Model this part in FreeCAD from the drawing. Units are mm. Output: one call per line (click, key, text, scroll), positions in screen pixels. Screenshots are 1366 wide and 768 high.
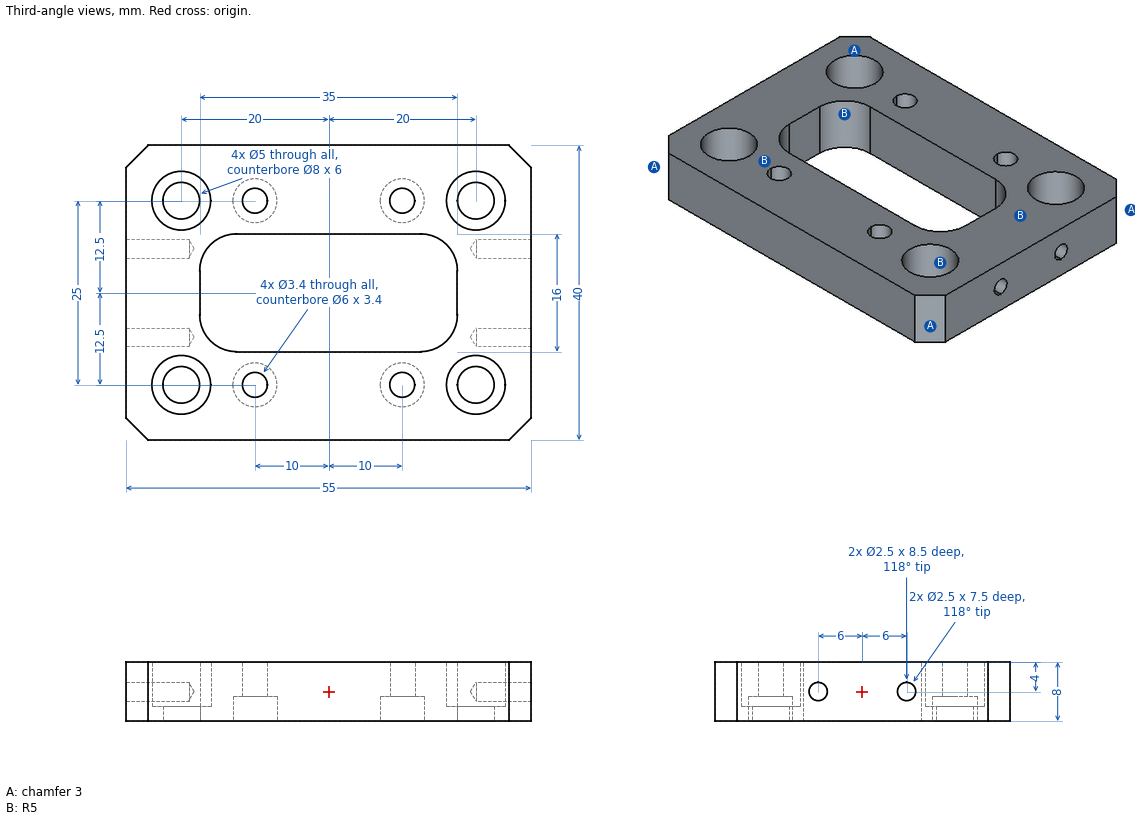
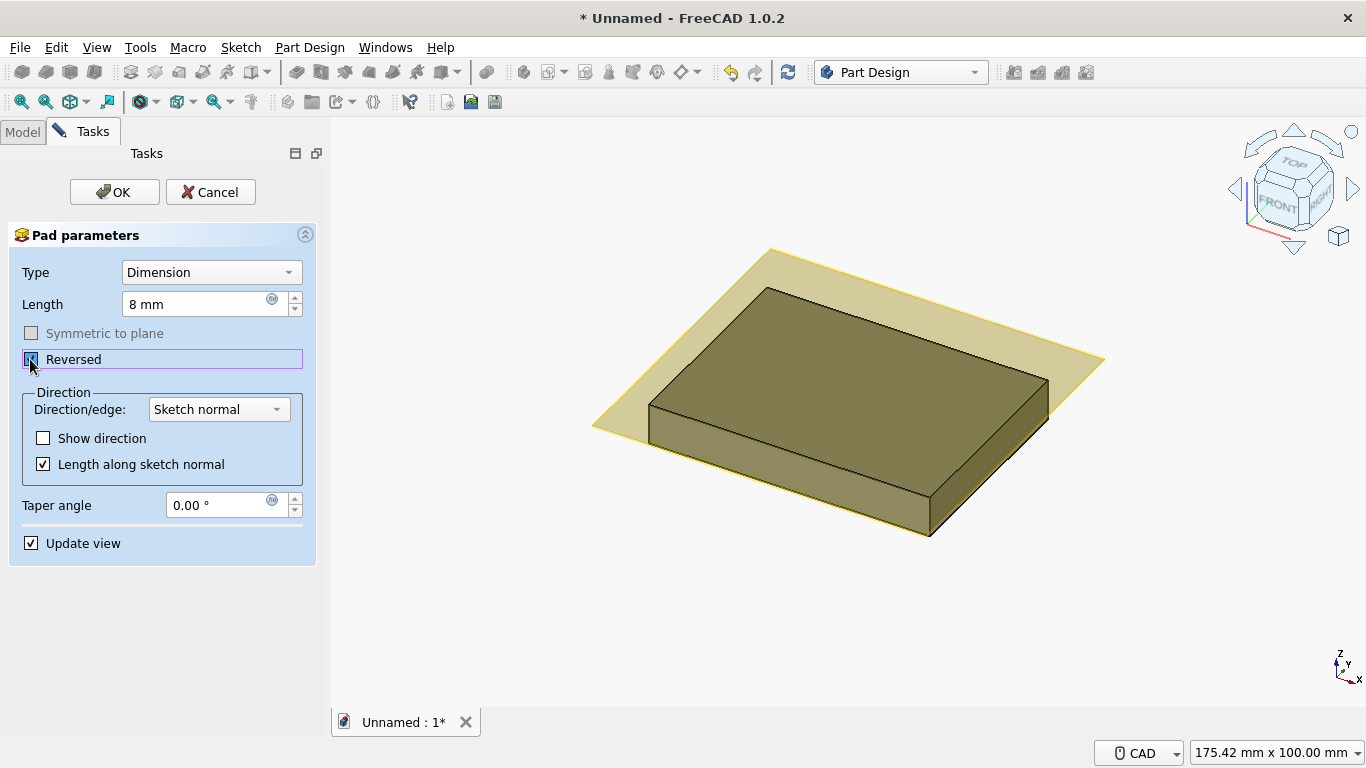
click(115, 192)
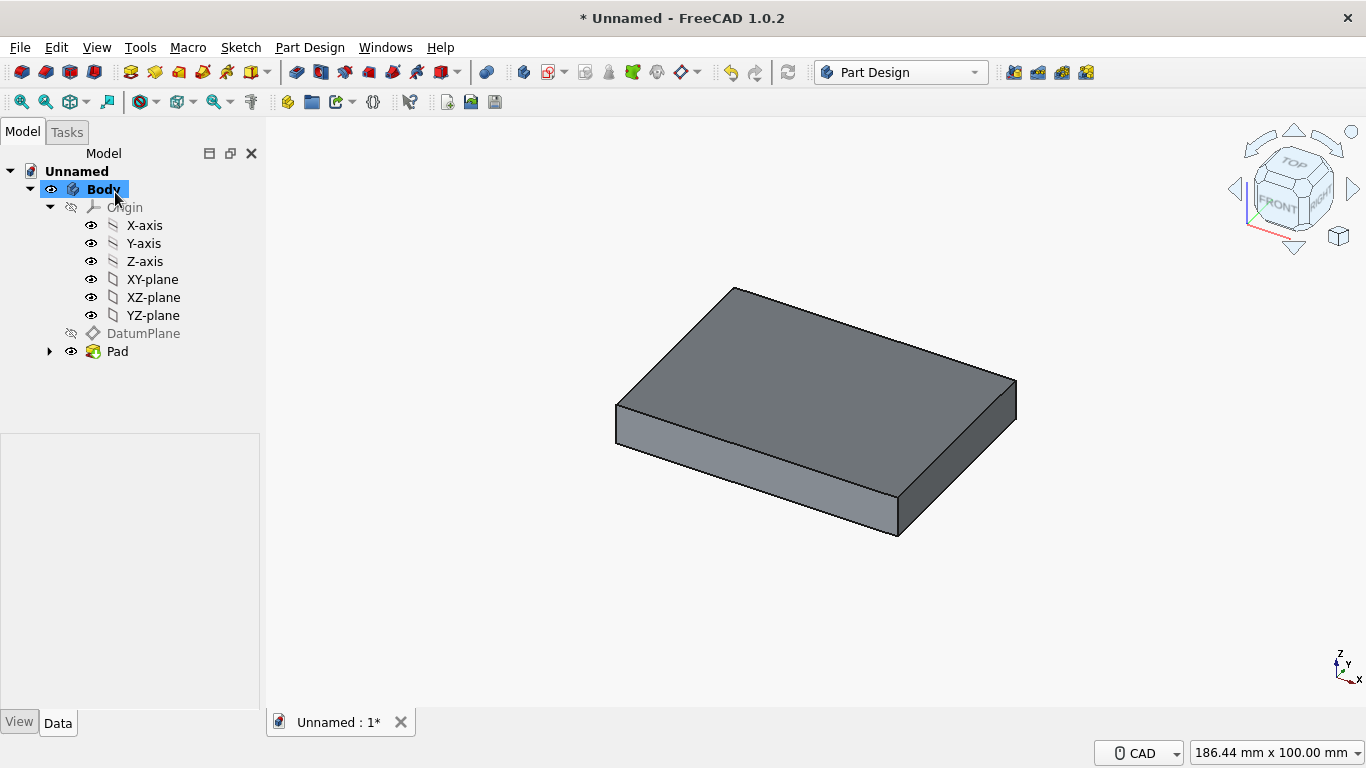
click(22, 102)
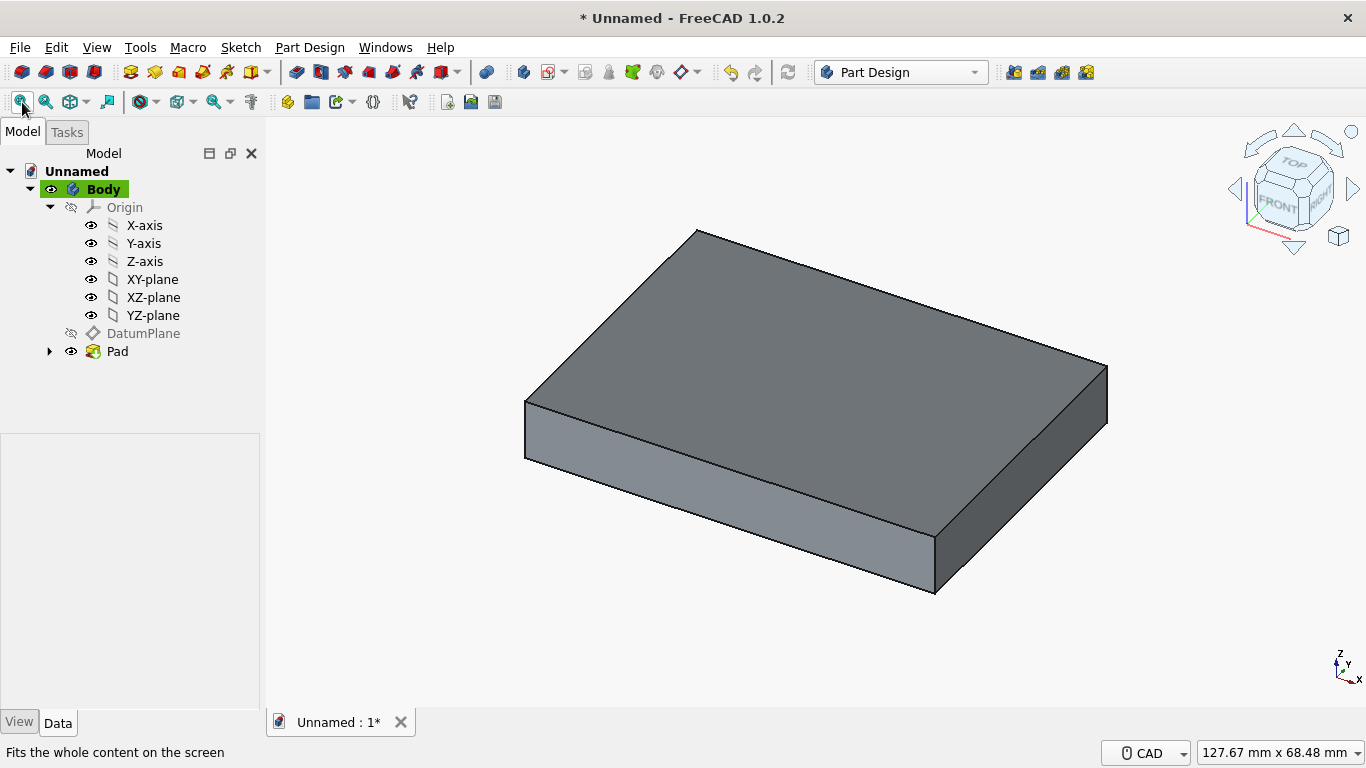
key(5)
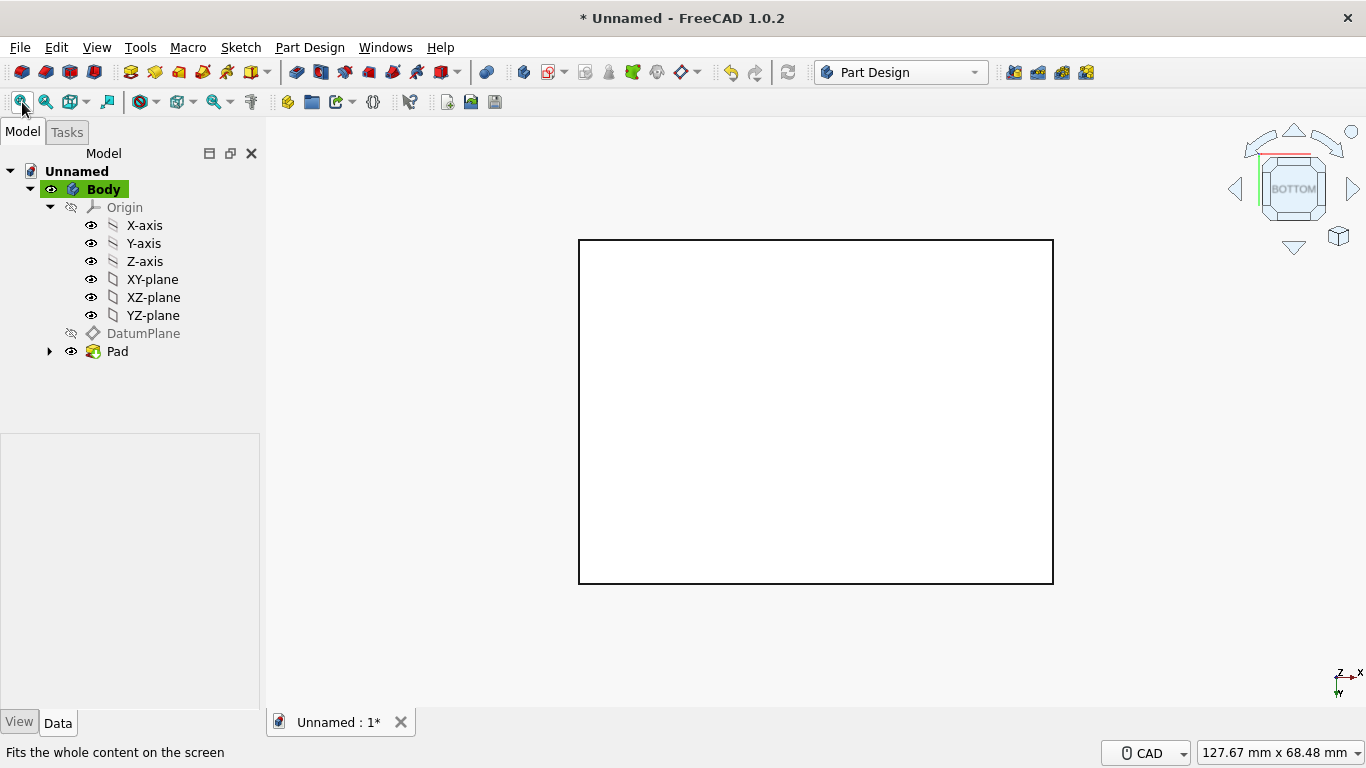
click(816, 411)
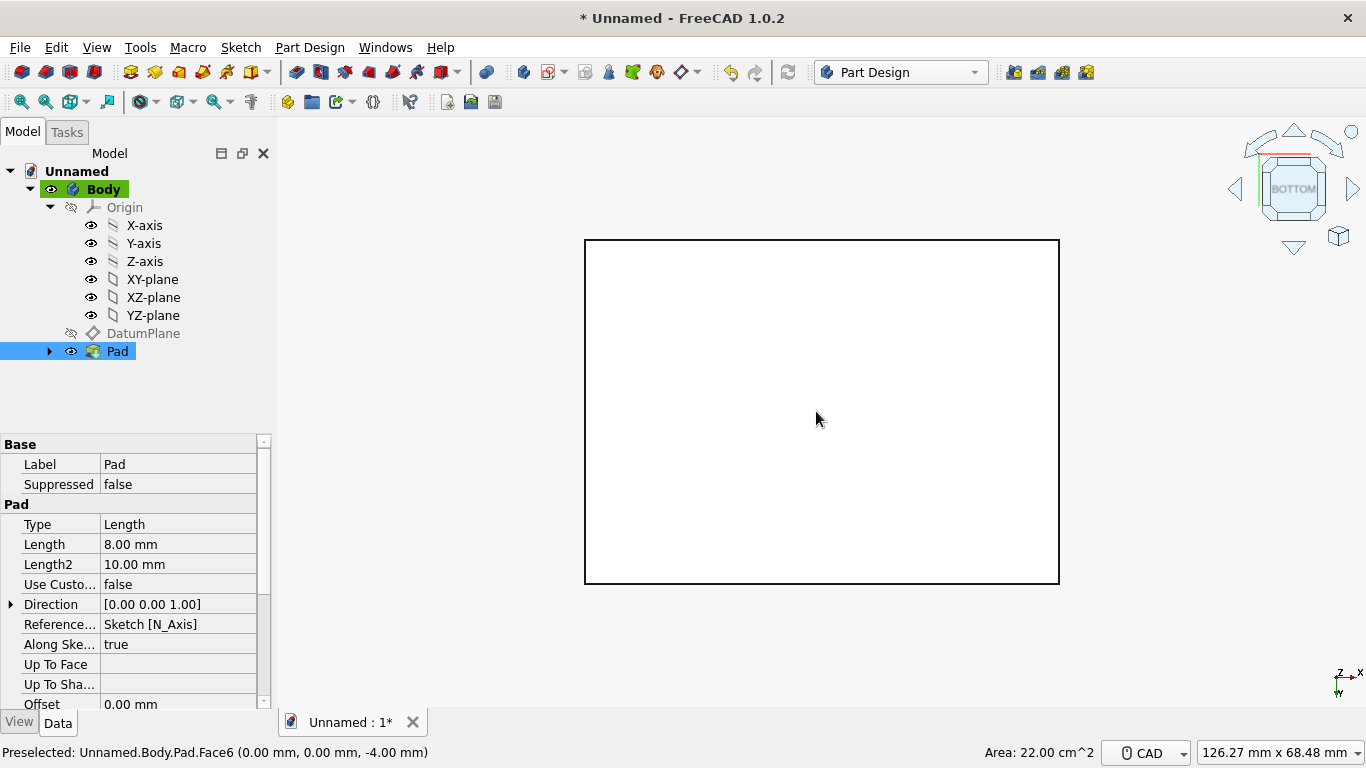
click(548, 72)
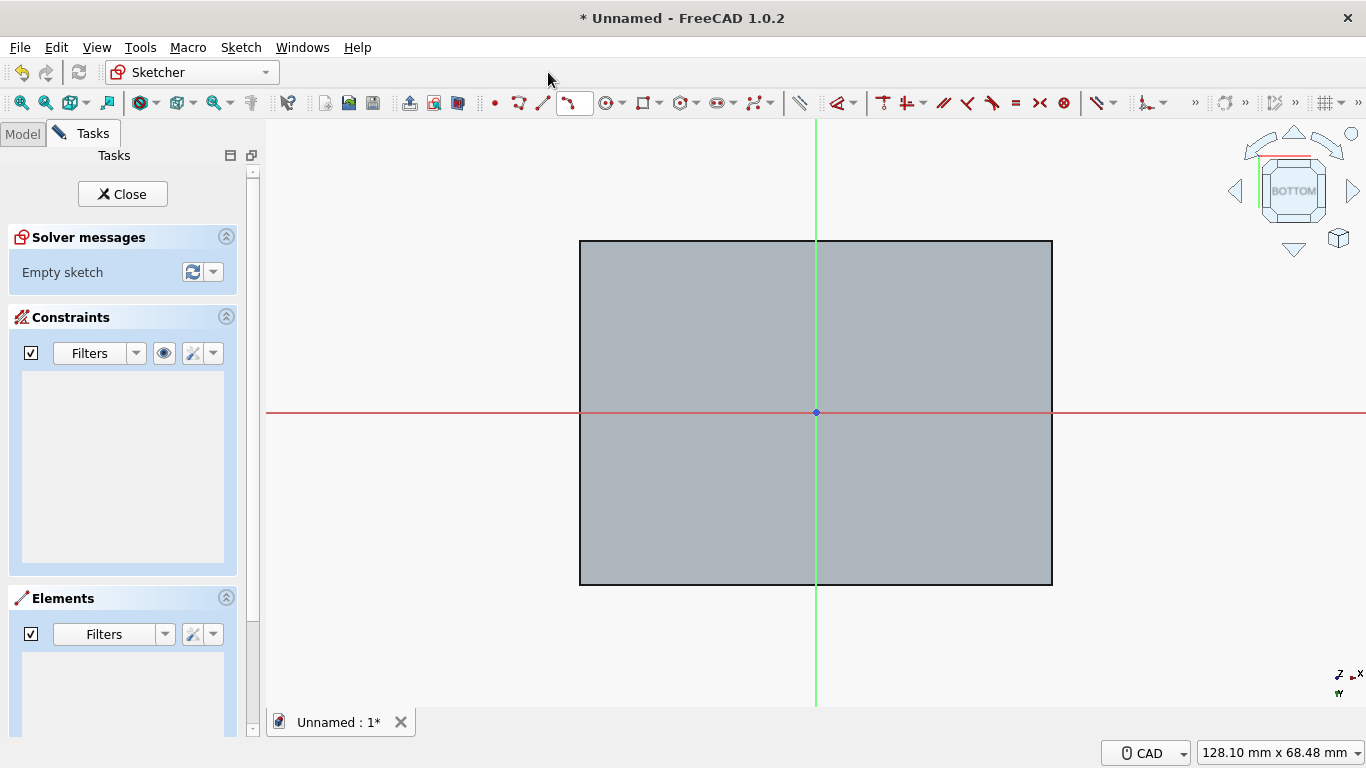
scroll(872, 413, up, 4)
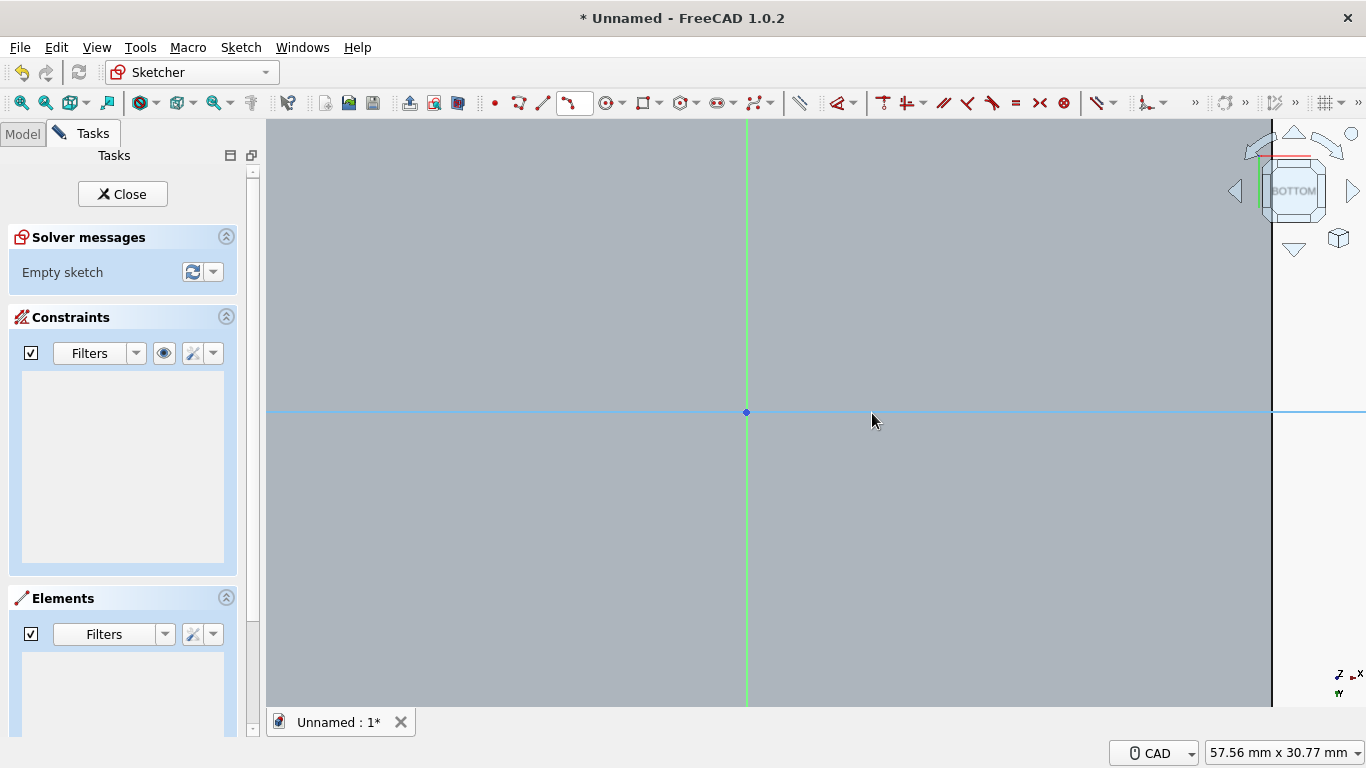
click(662, 104)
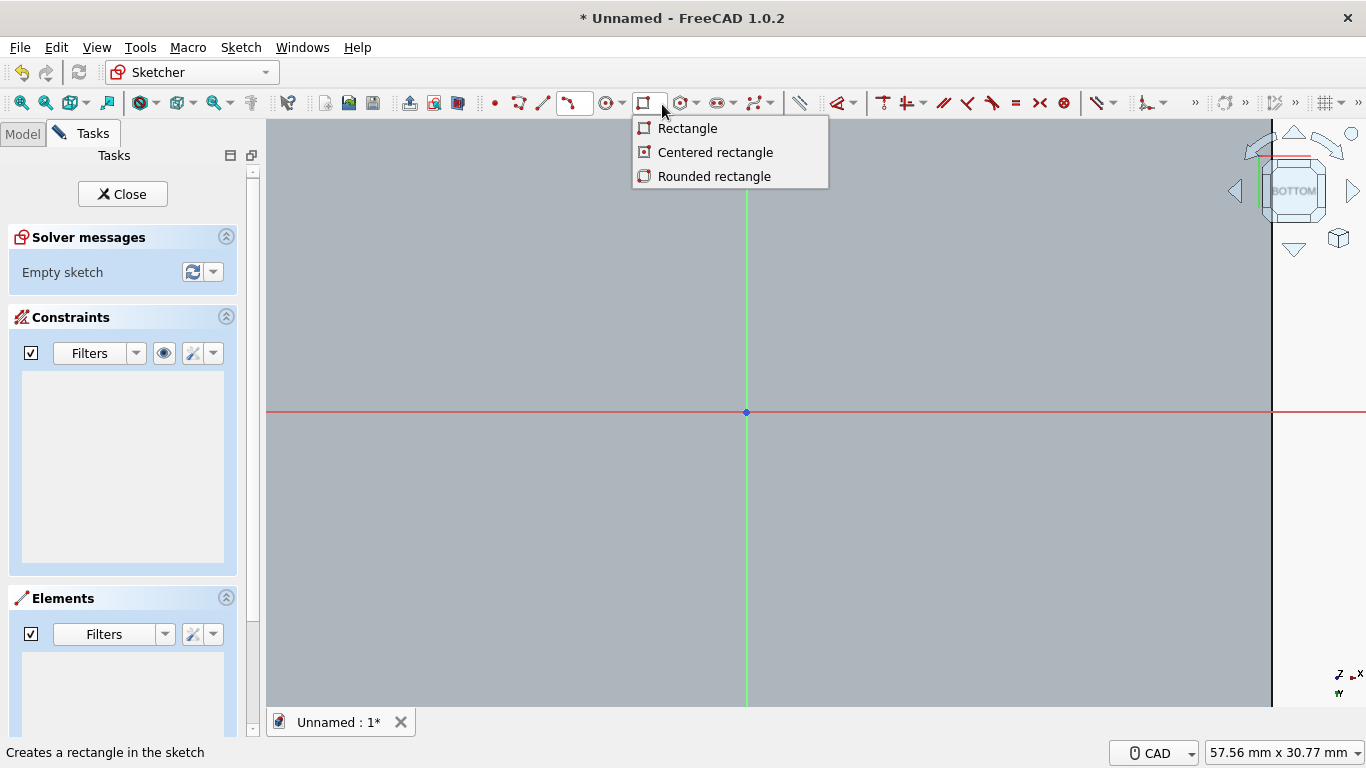
click(730, 152)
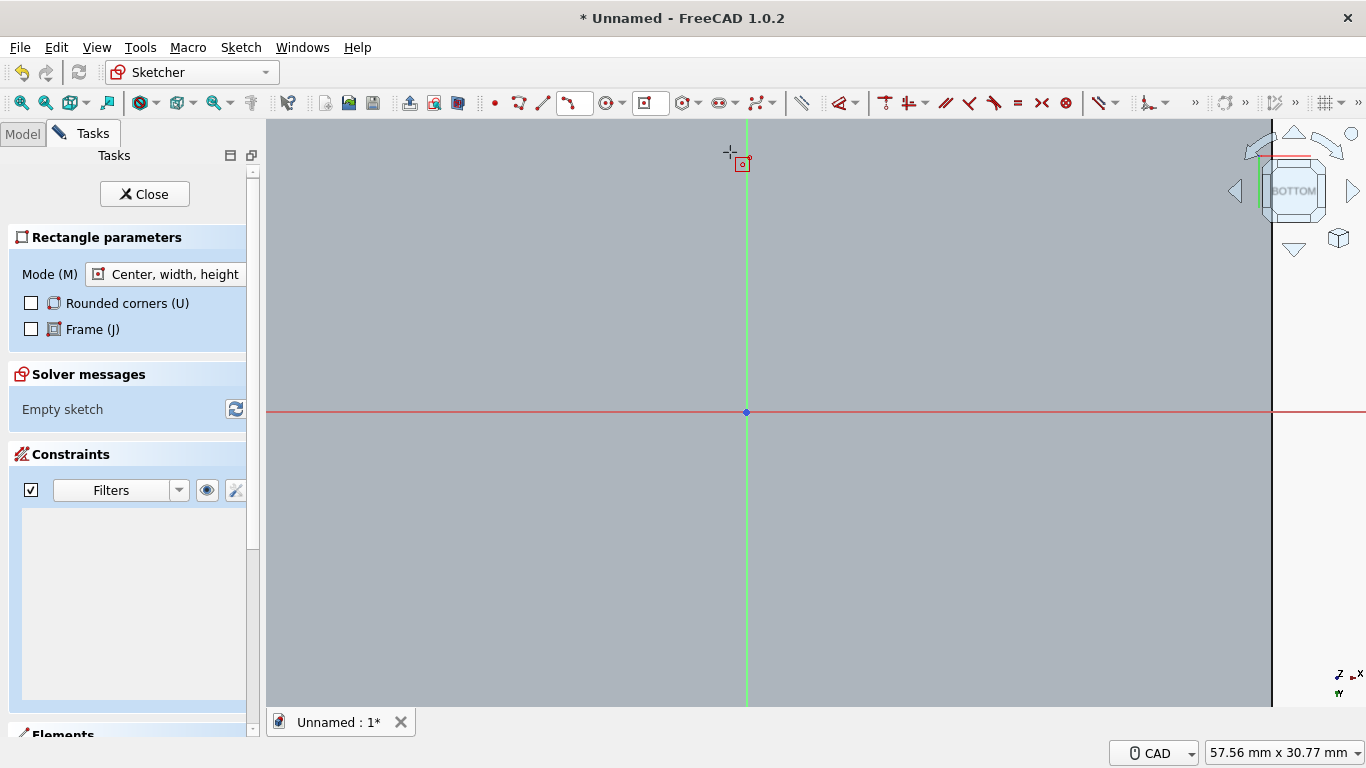
click(747, 412)
move(1081, 260)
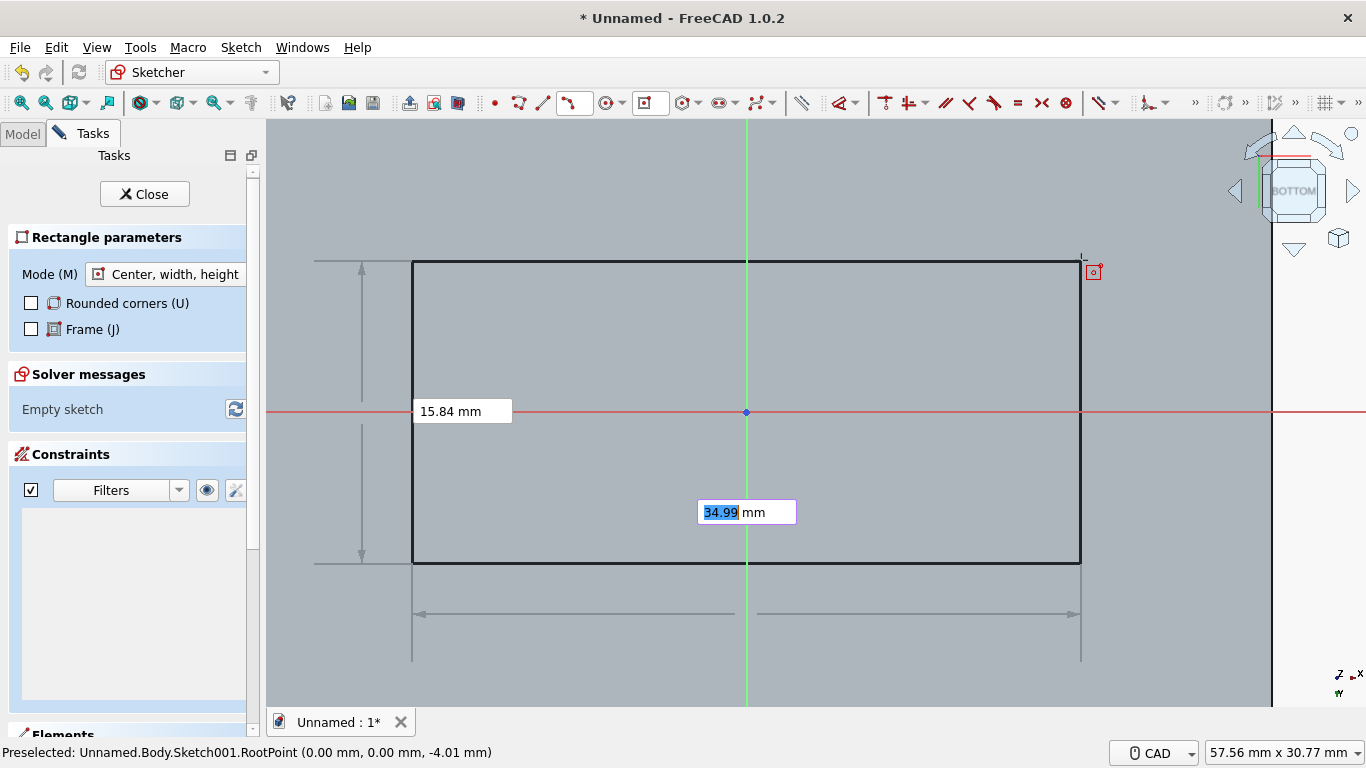
text(35)
key(Tab)
text(16)
key(Return)
key(Escape)